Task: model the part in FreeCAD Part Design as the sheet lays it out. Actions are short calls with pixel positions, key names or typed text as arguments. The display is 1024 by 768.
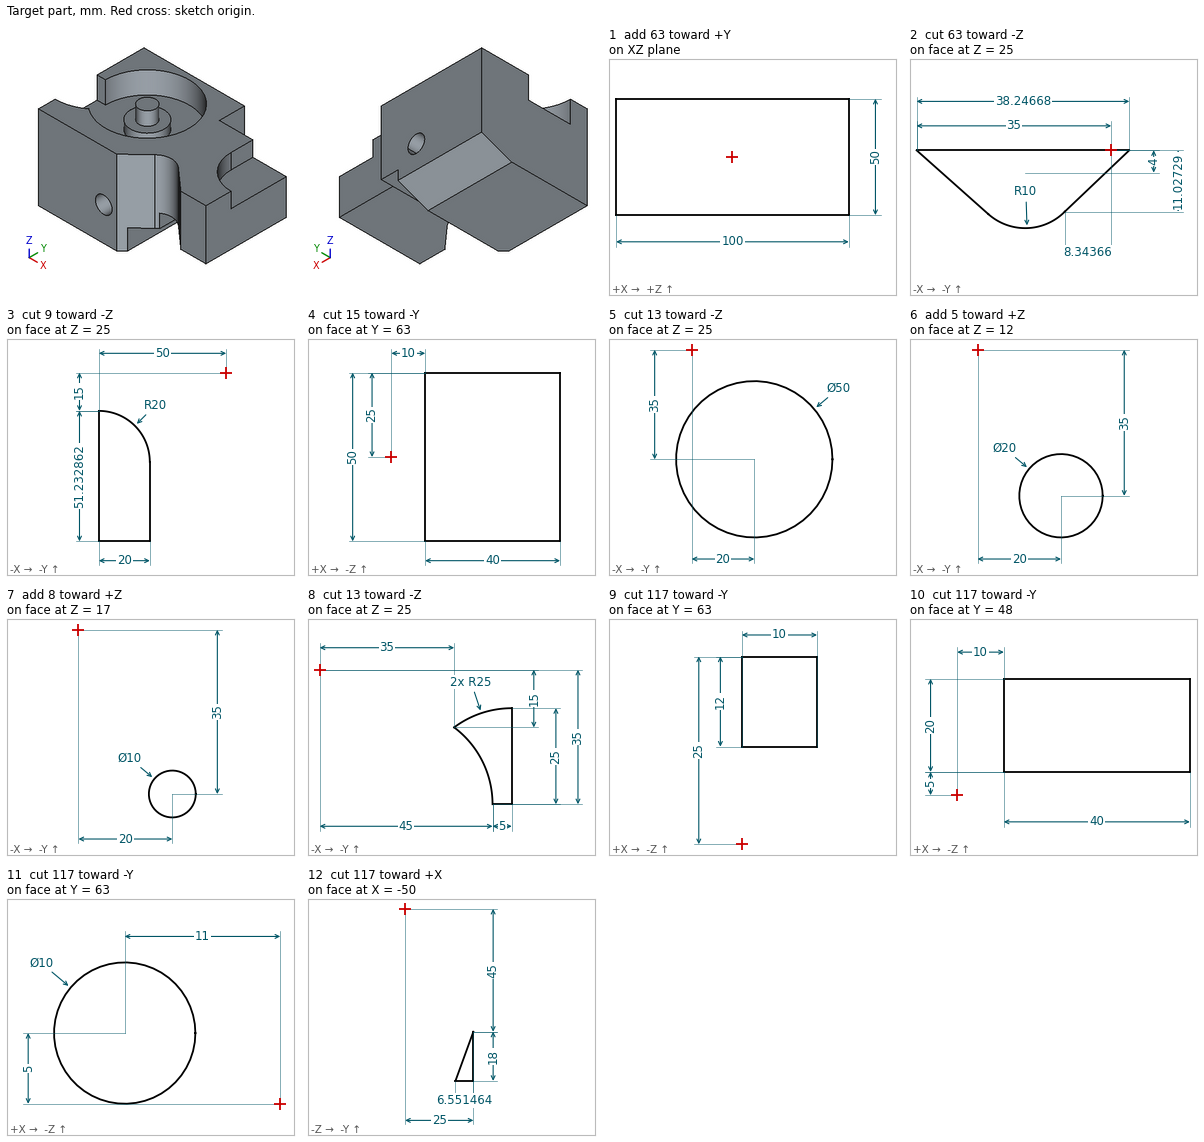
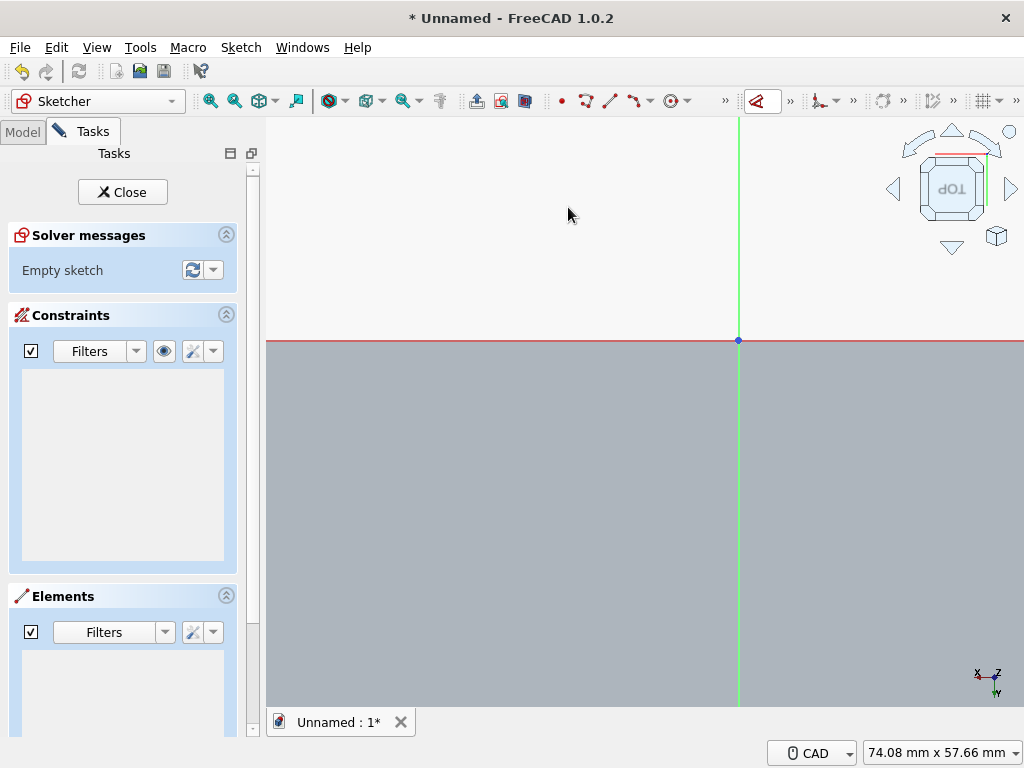
click(586, 102)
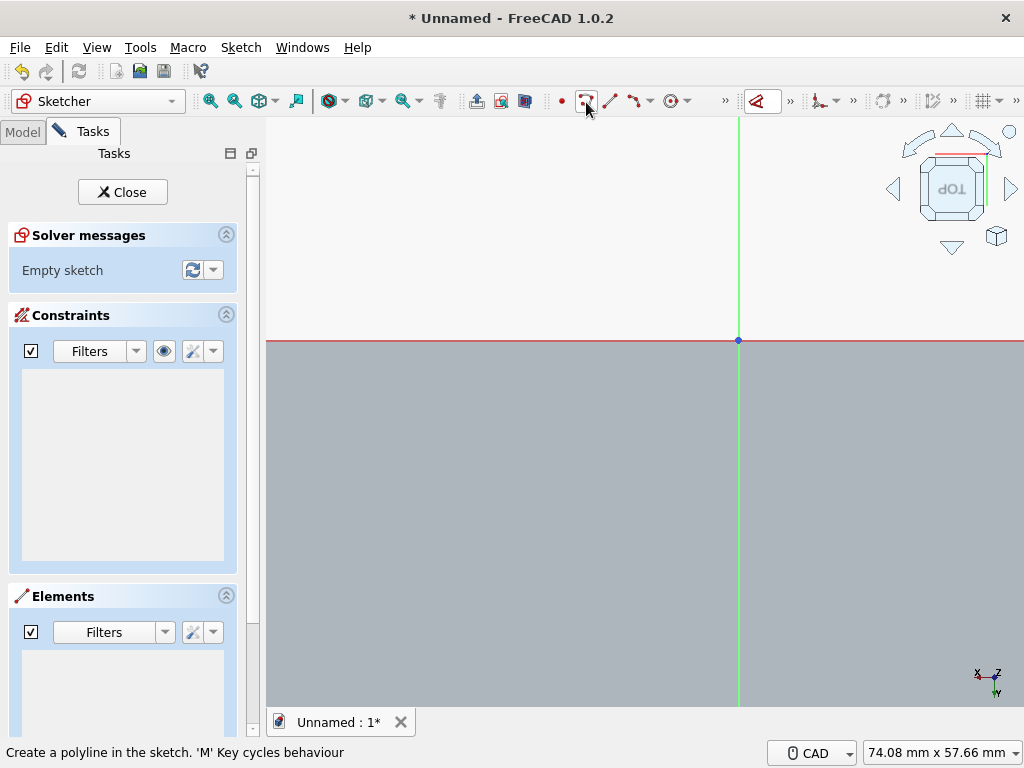
click(654, 454)
click(772, 341)
click(381, 350)
click(513, 458)
right_click(513, 458)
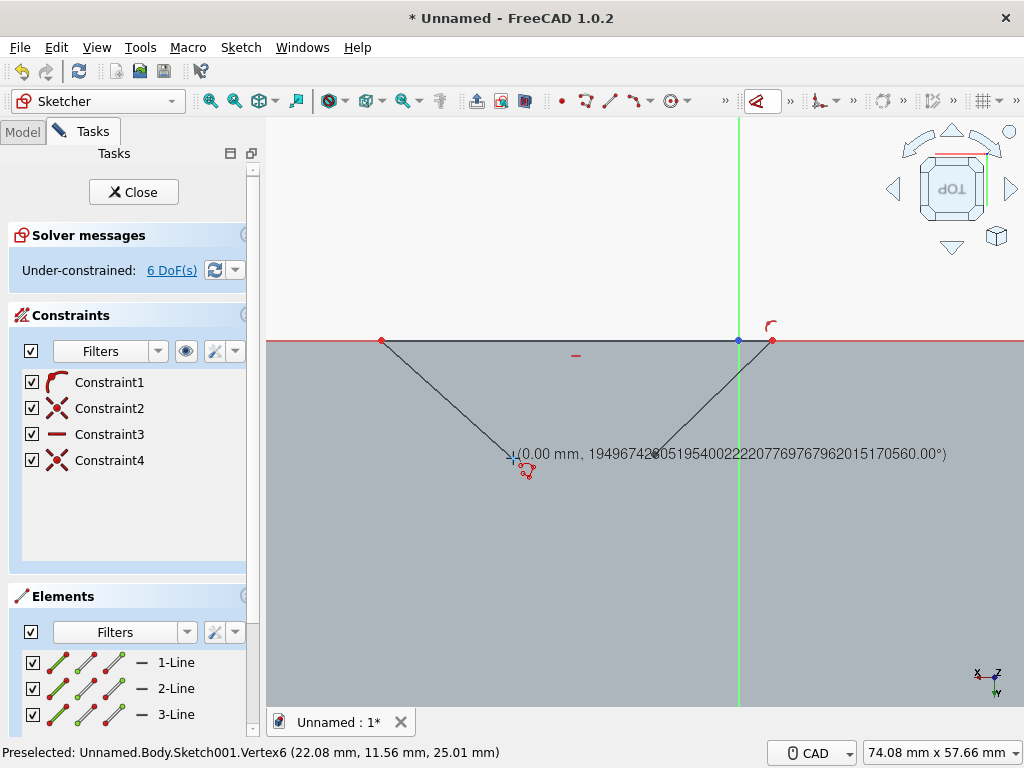
click(634, 102)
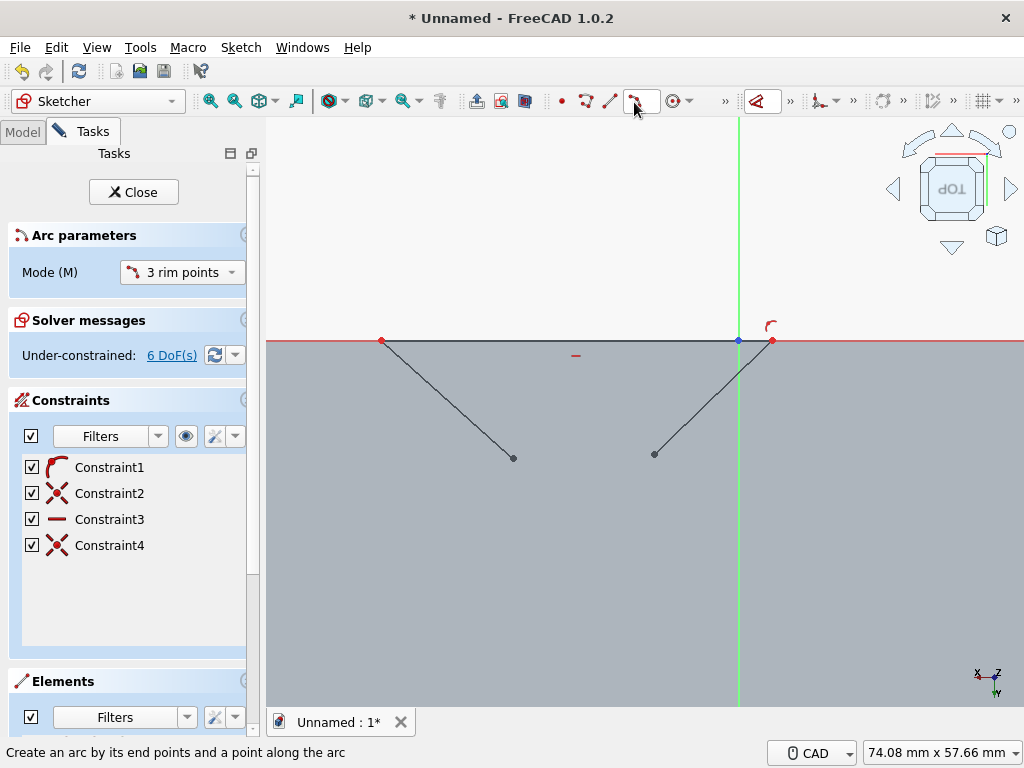
click(513, 459)
click(654, 455)
click(584, 484)
key(Escape)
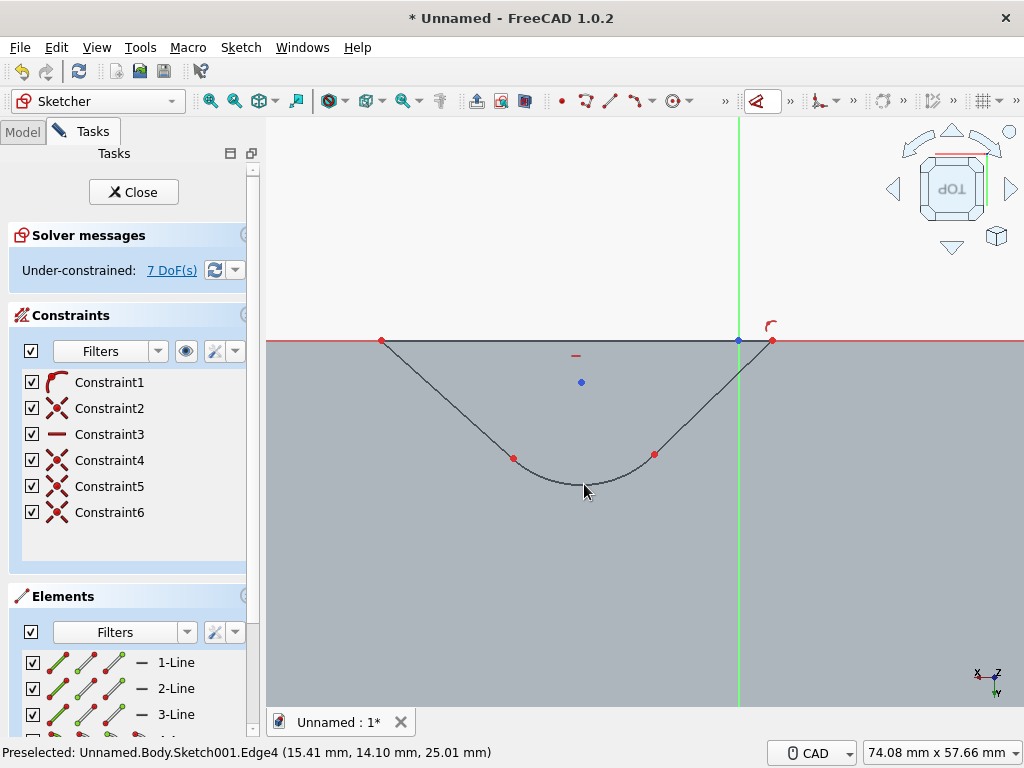
click(421, 376)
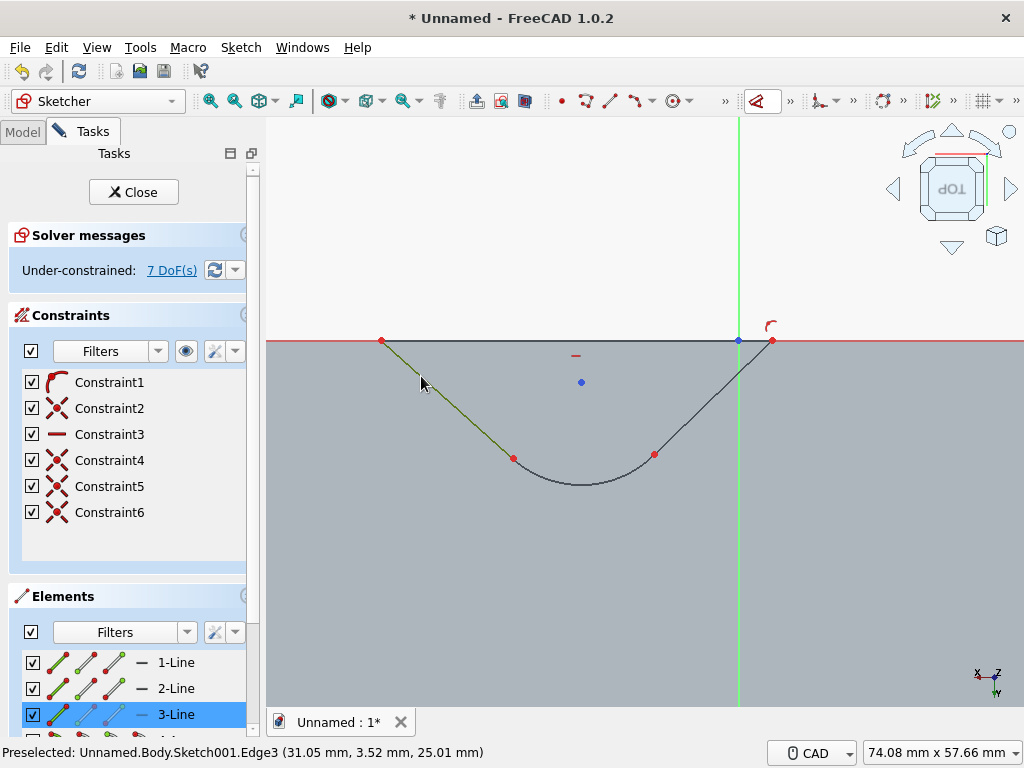
click(554, 481)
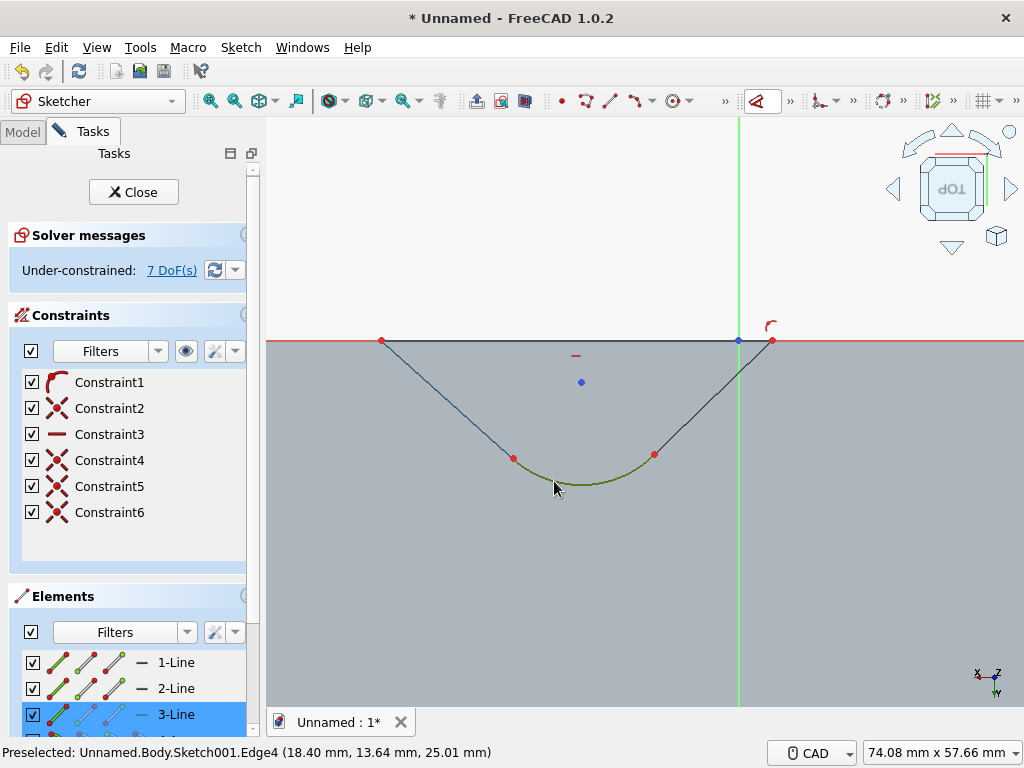
key(t)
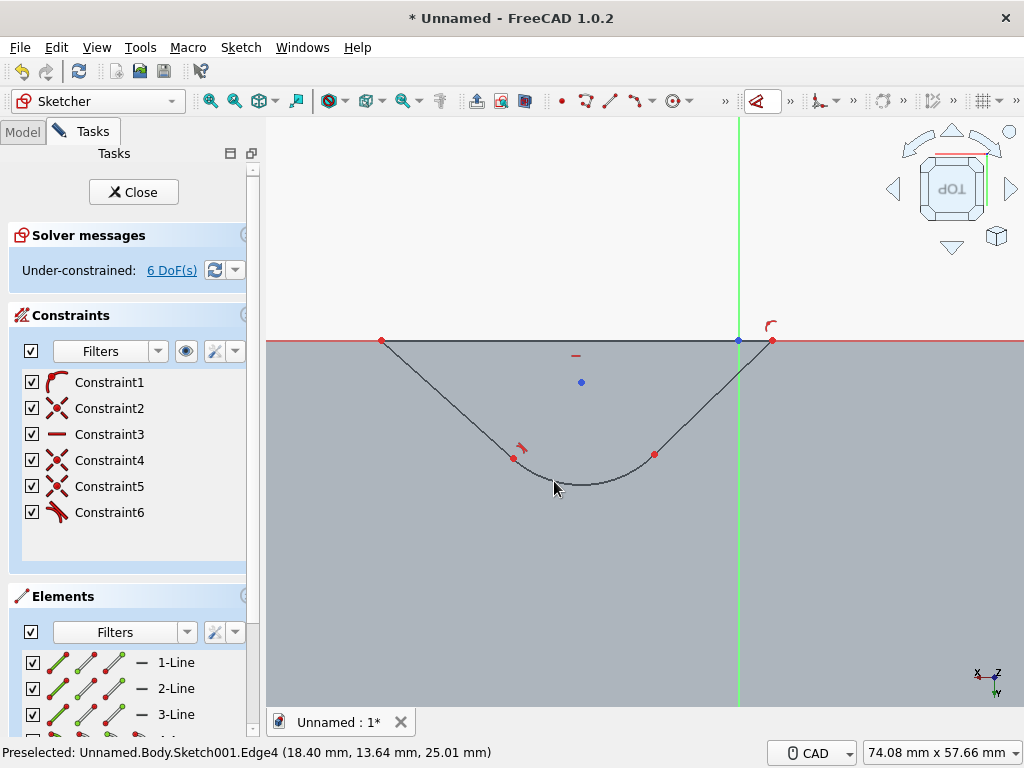
click(554, 481)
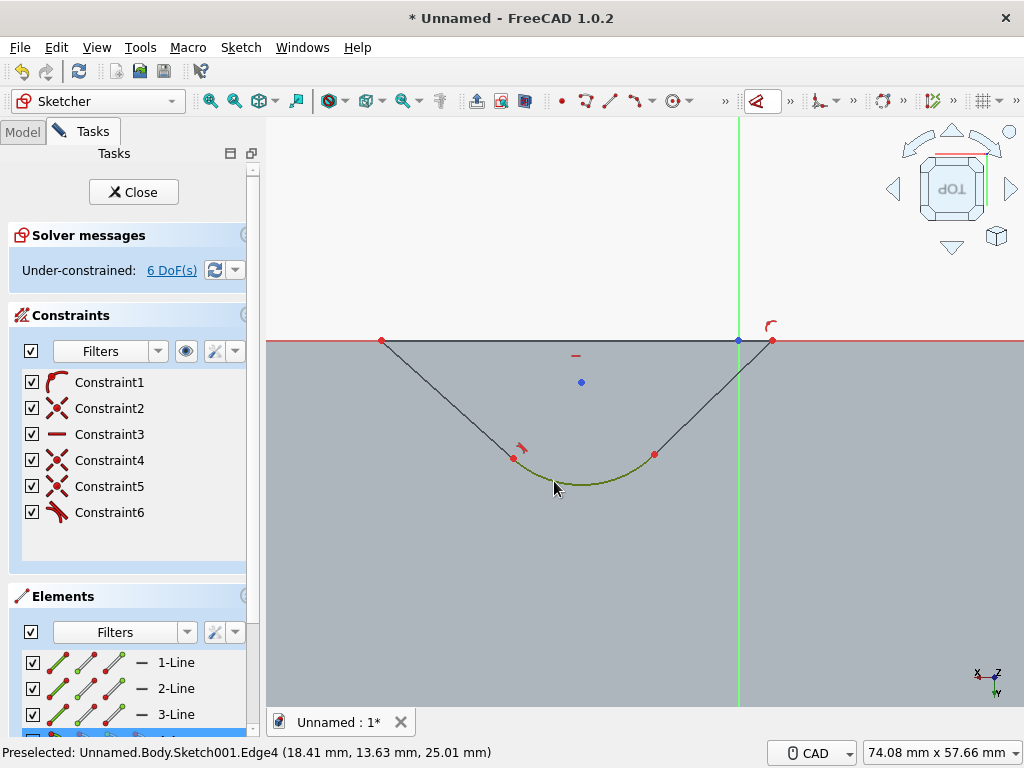
click(776, 102)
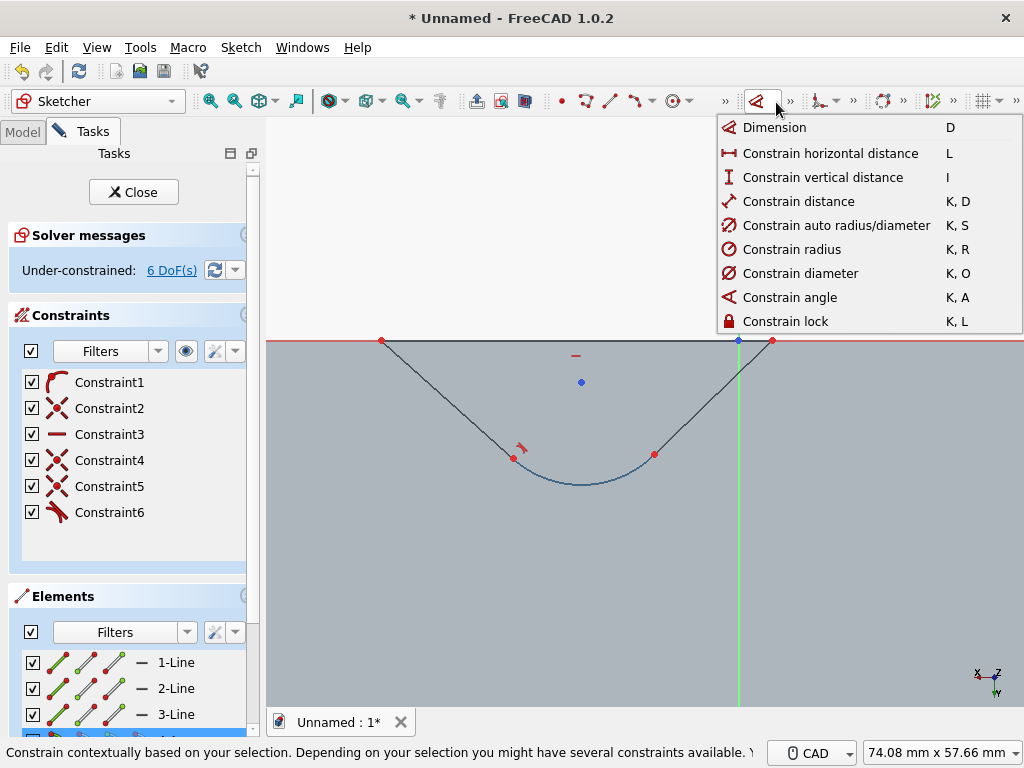
click(870, 249)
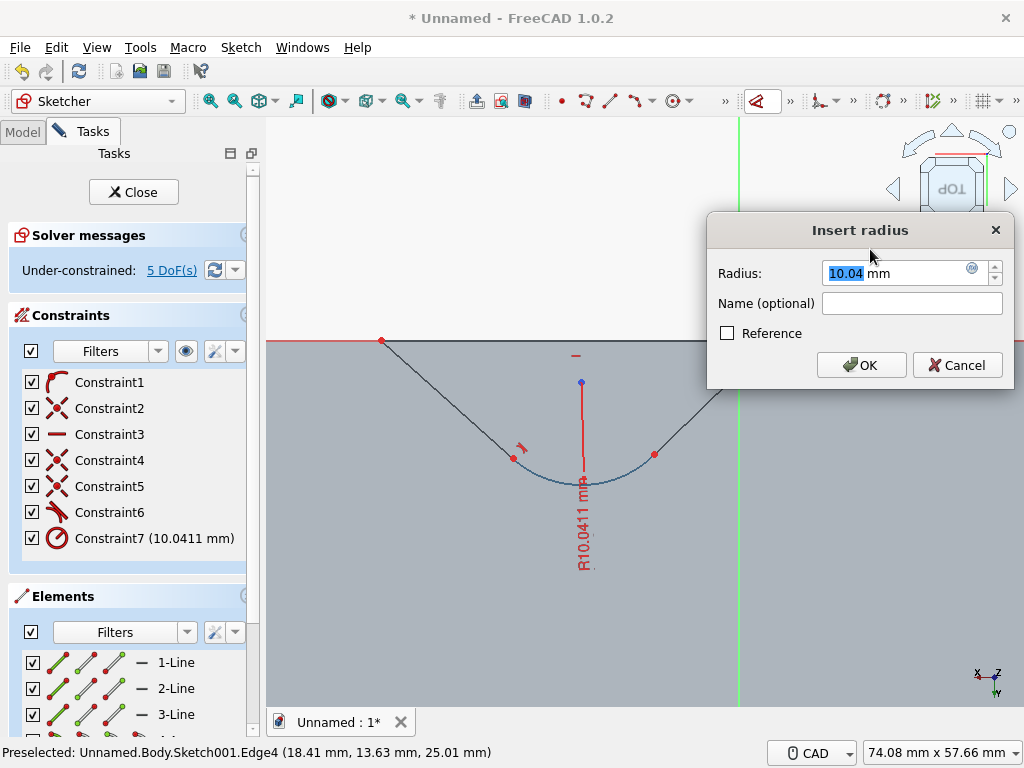
text(10)
key(Return)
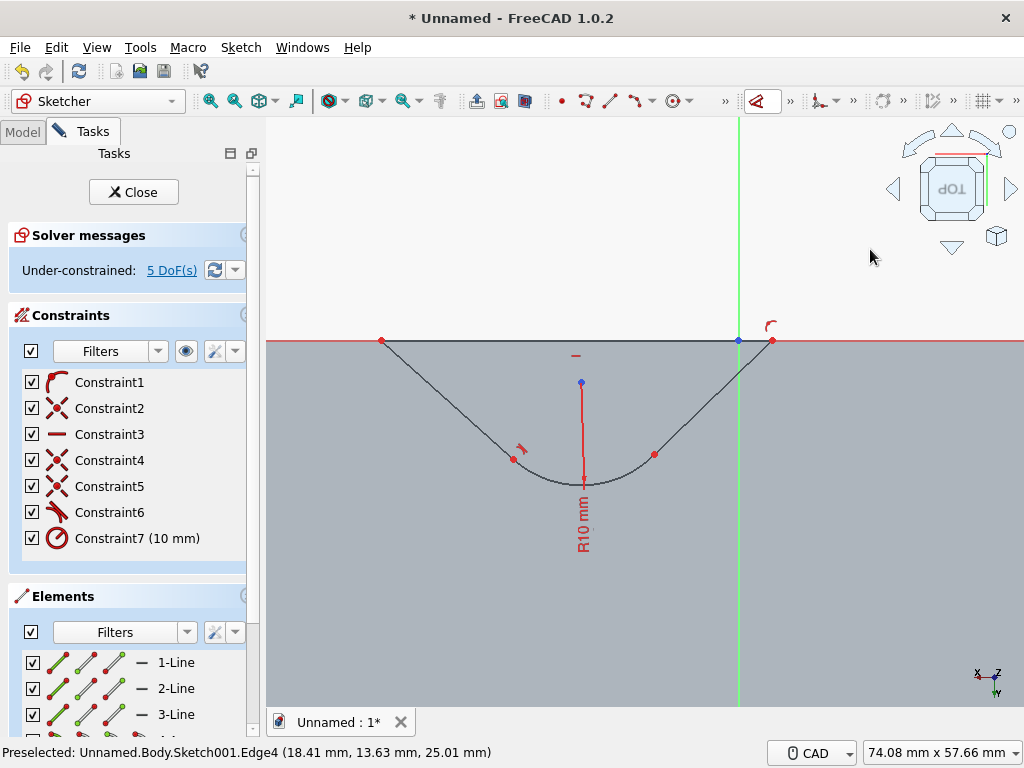
click(581, 383)